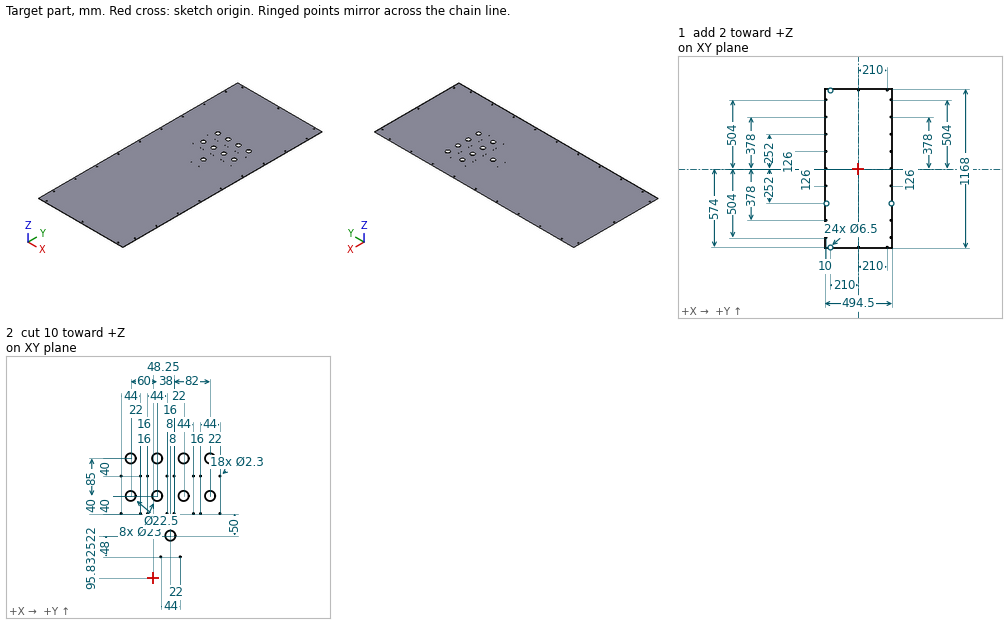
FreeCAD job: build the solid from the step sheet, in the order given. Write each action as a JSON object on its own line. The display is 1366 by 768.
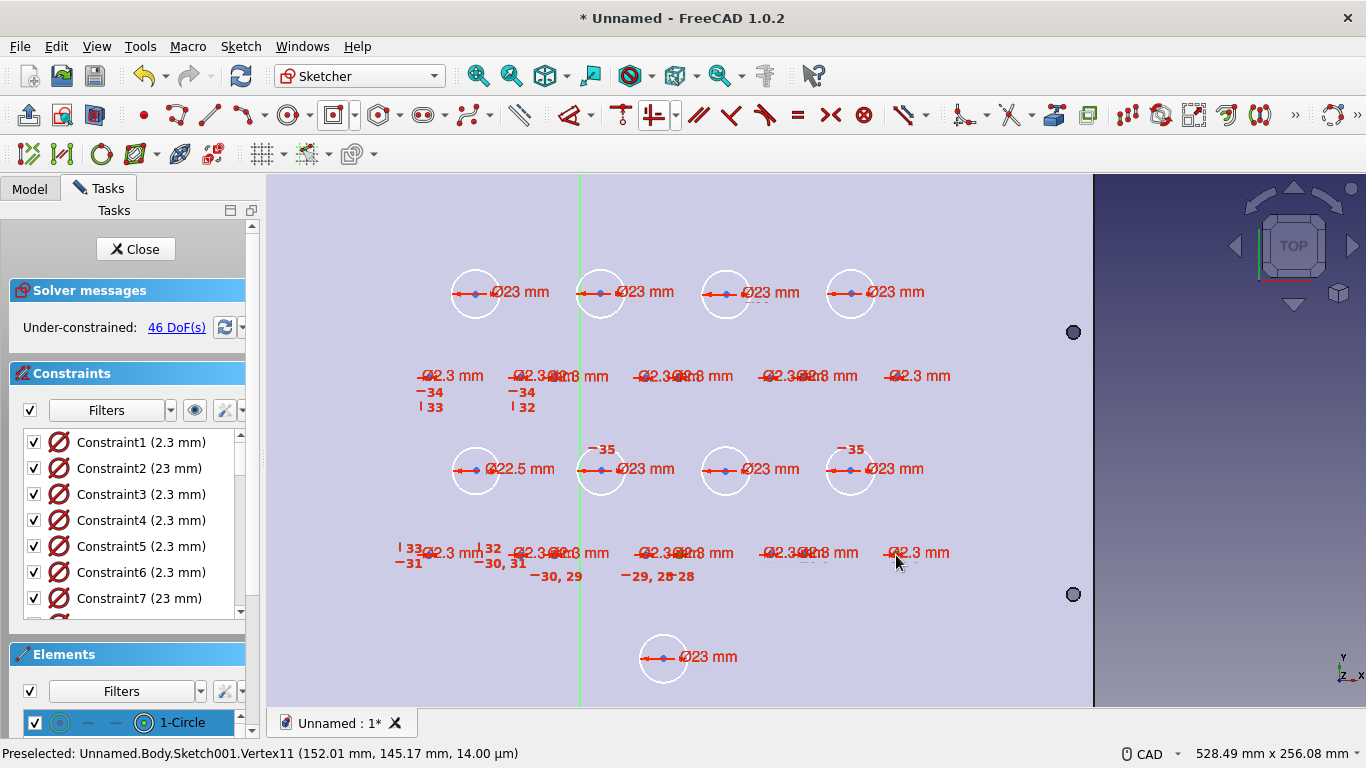
{"action": "left_click", "coordinate": [676, 116]}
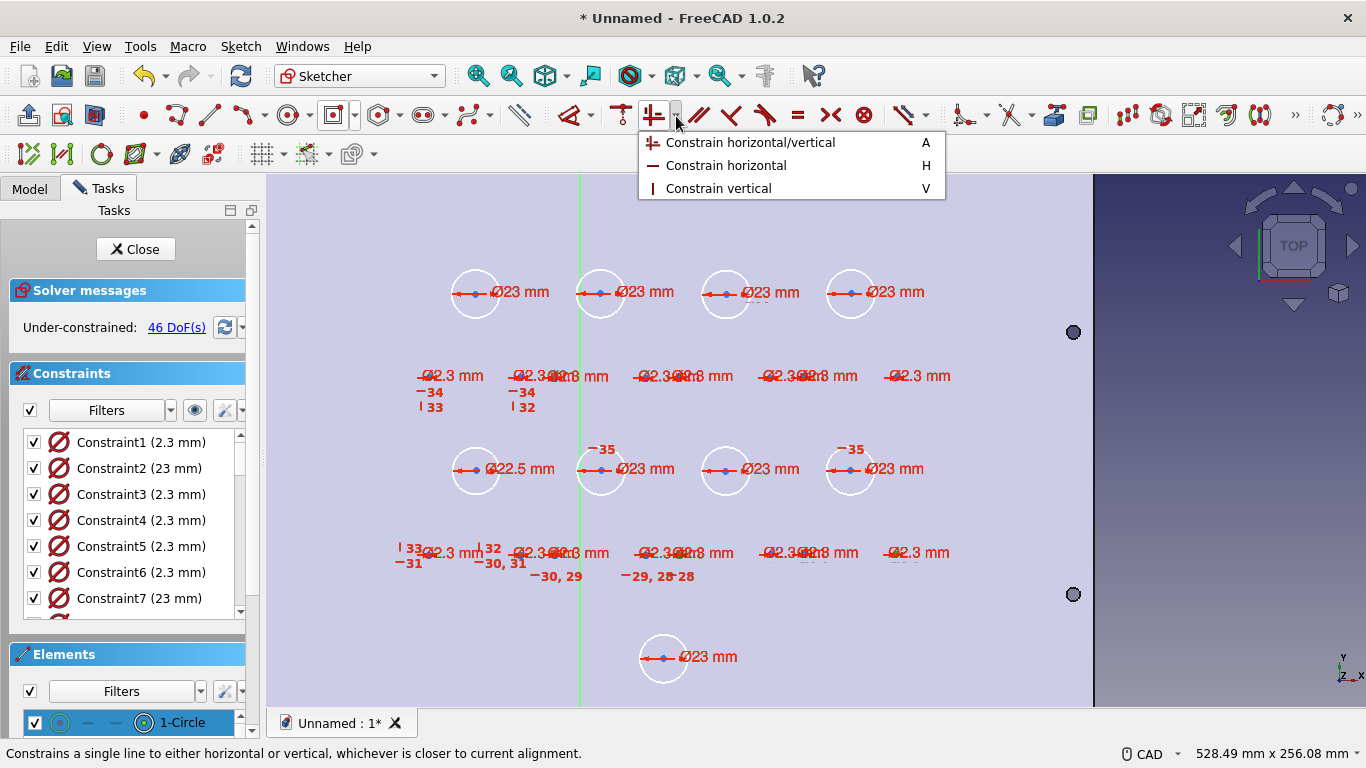
{"action": "left_click", "coordinate": [792, 166]}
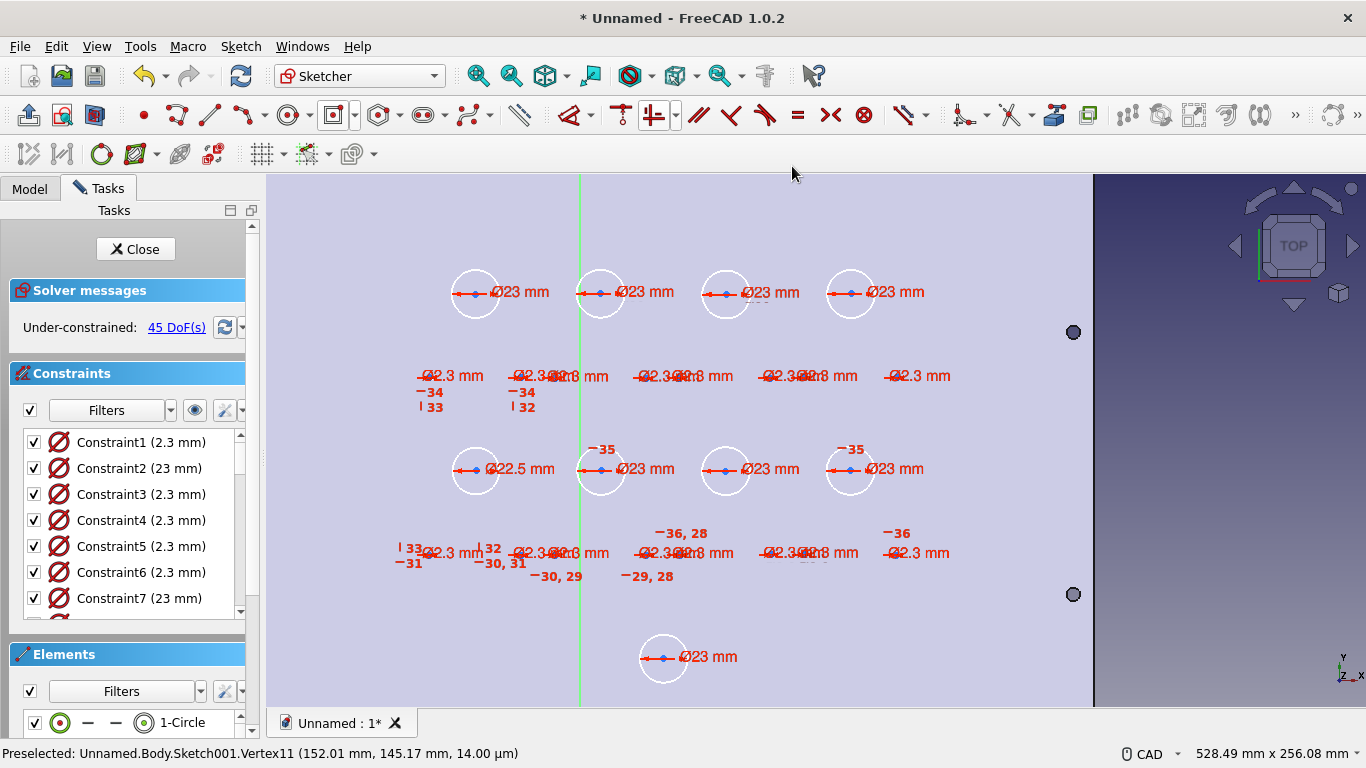
{"action": "left_click", "coordinate": [896, 555]}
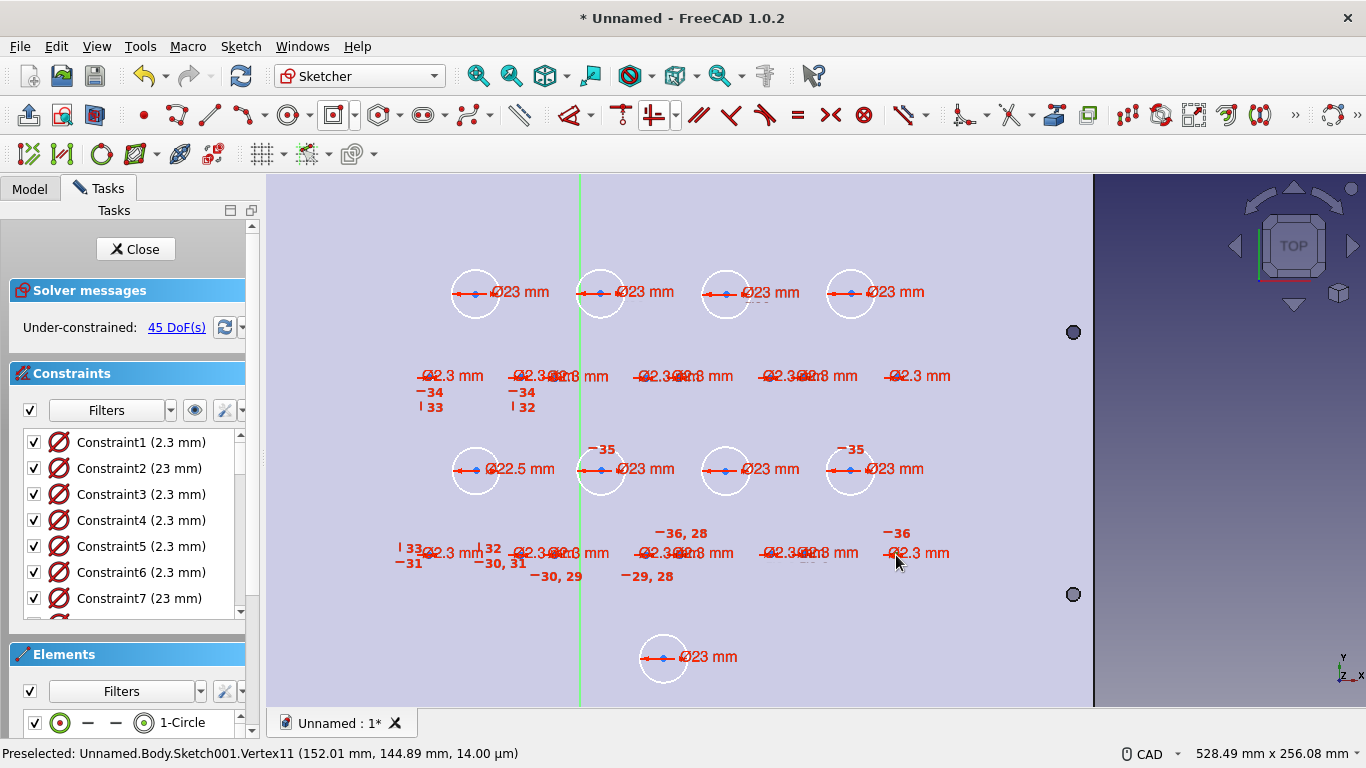
{"action": "left_click", "coordinate": [805, 555]}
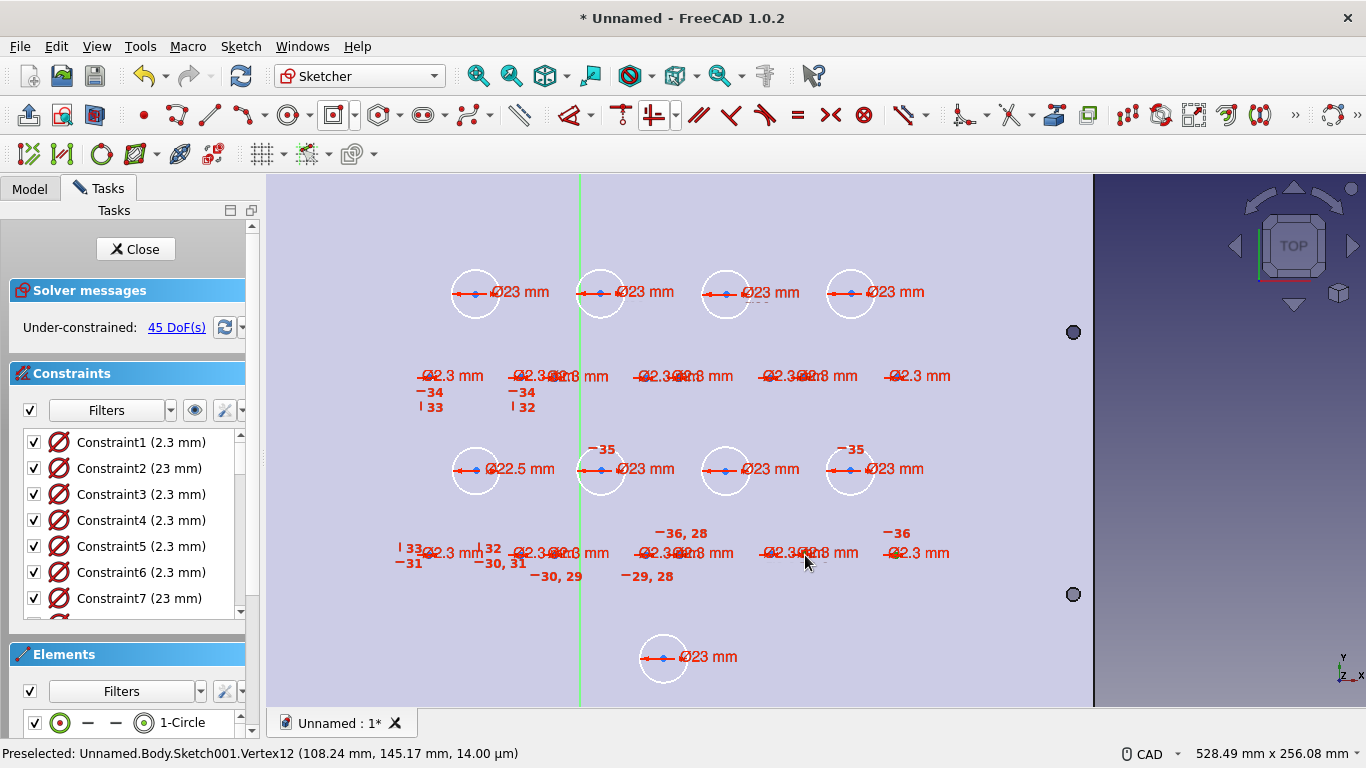
{"action": "left_click", "coordinate": [676, 116]}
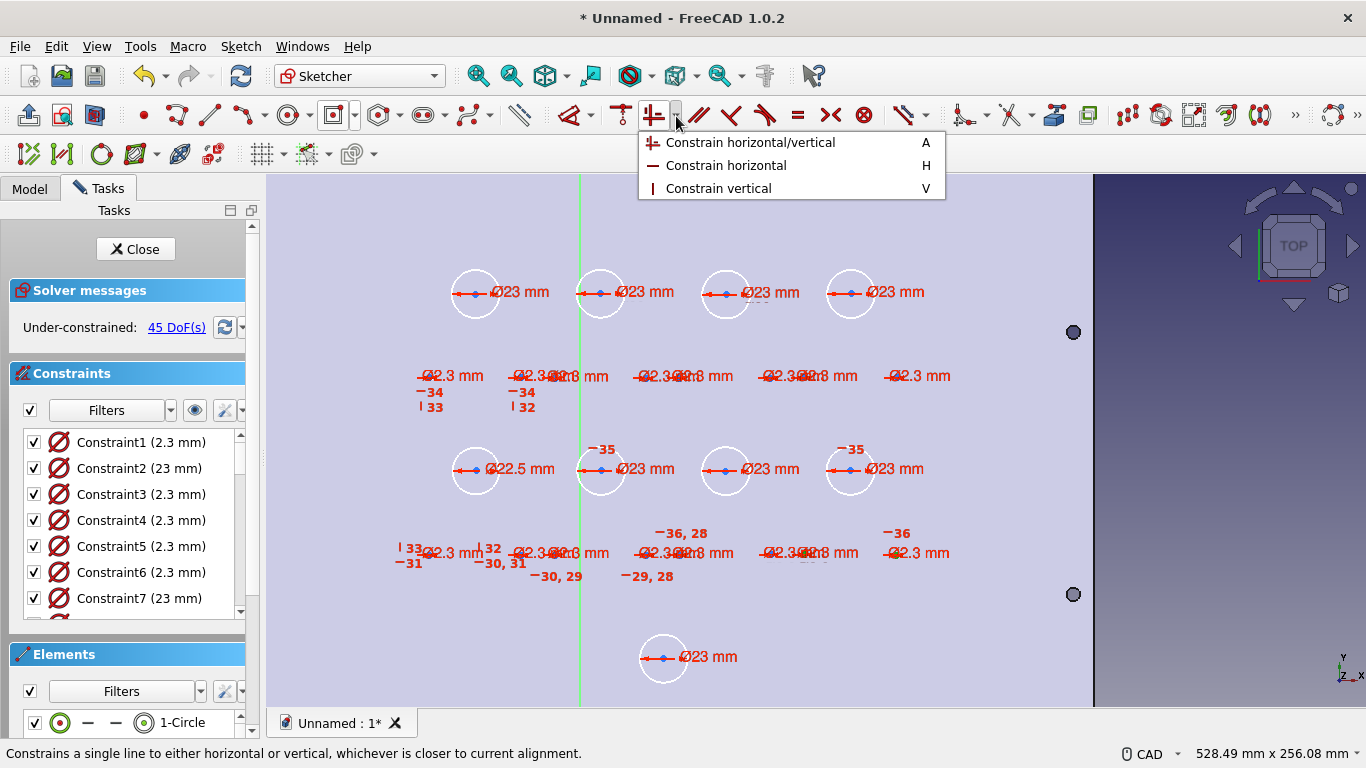
{"action": "left_click", "coordinate": [792, 166]}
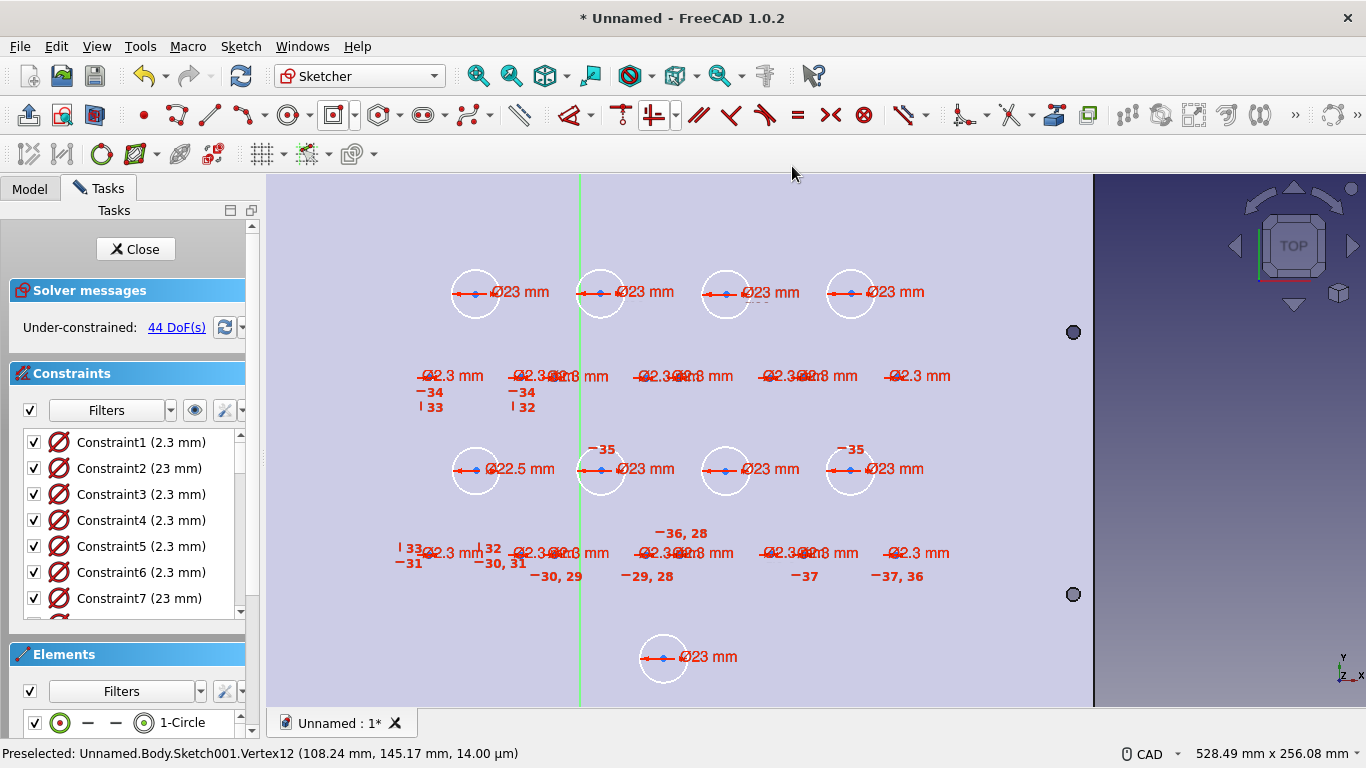
{"action": "left_click", "coordinate": [601, 471]}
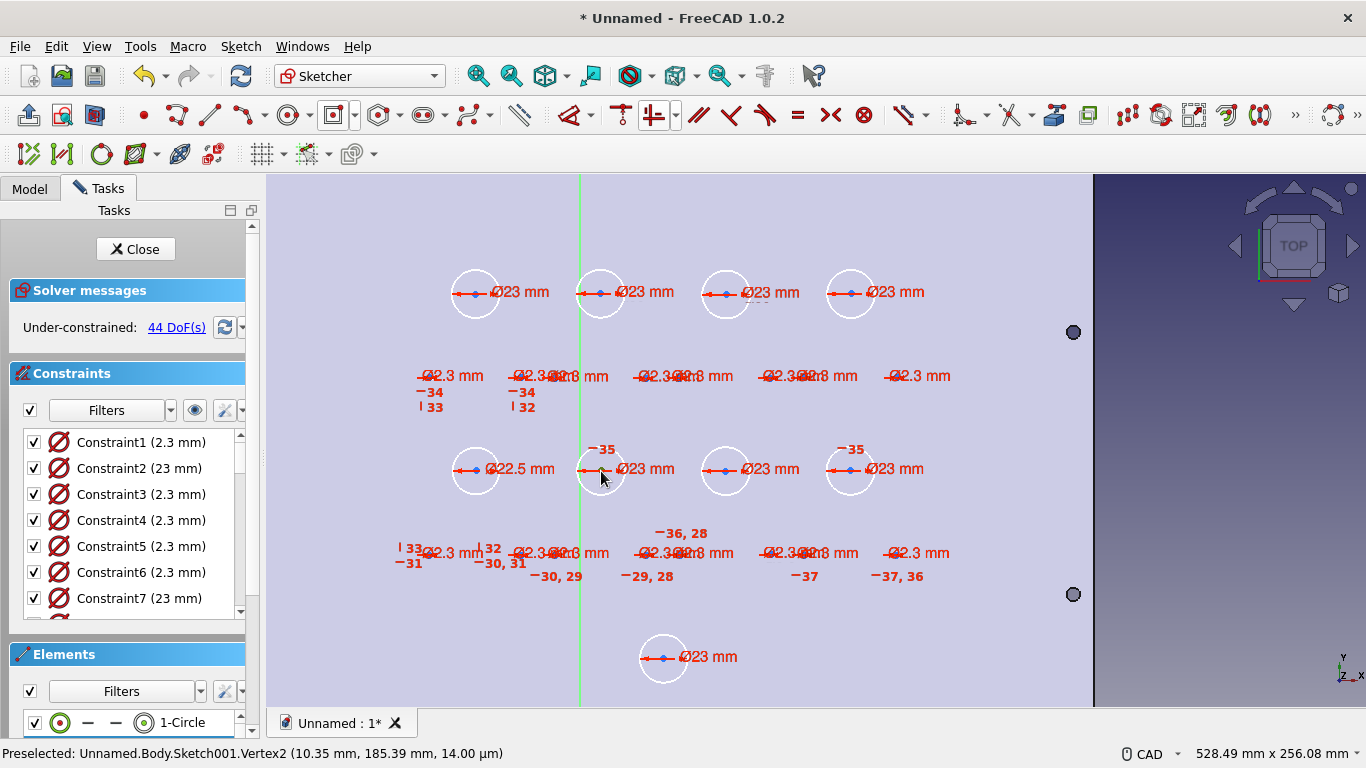
{"action": "left_click", "coordinate": [726, 471]}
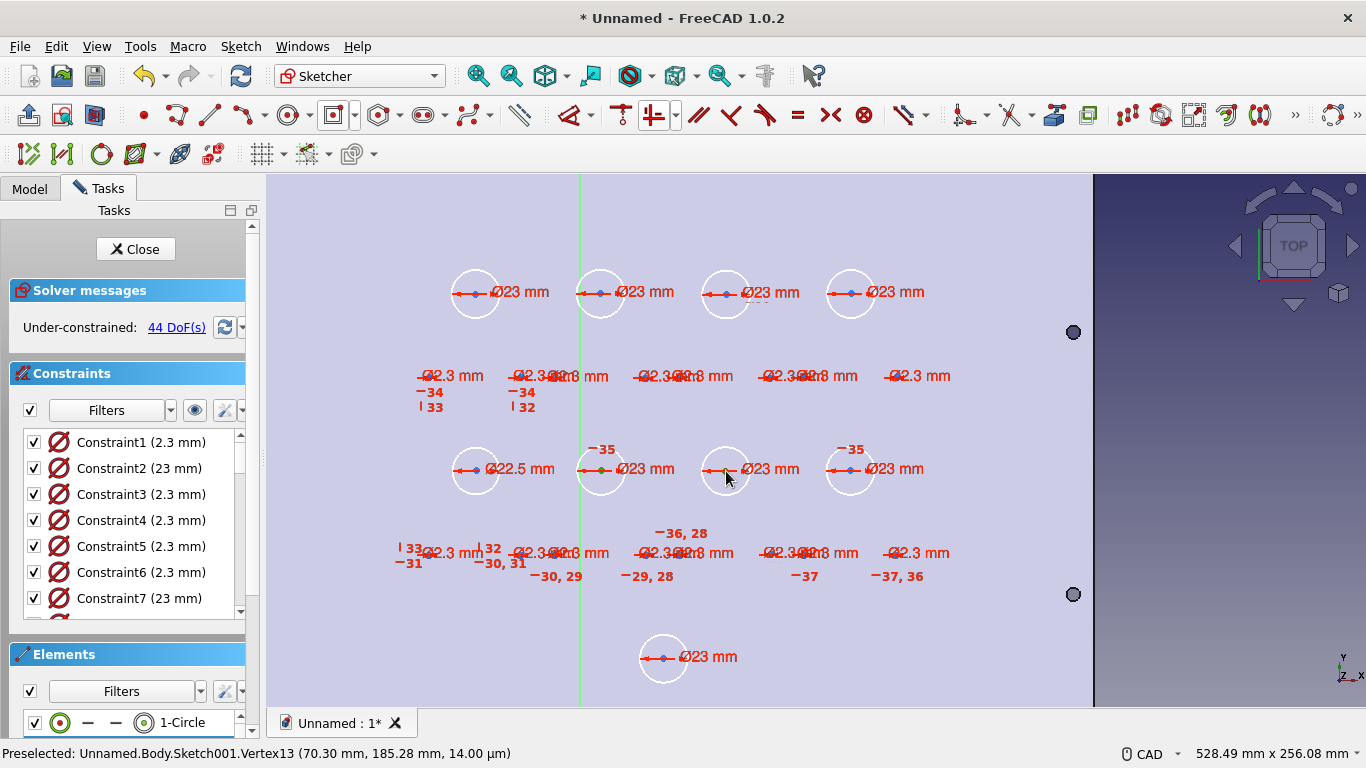
{"action": "left_click", "coordinate": [676, 116]}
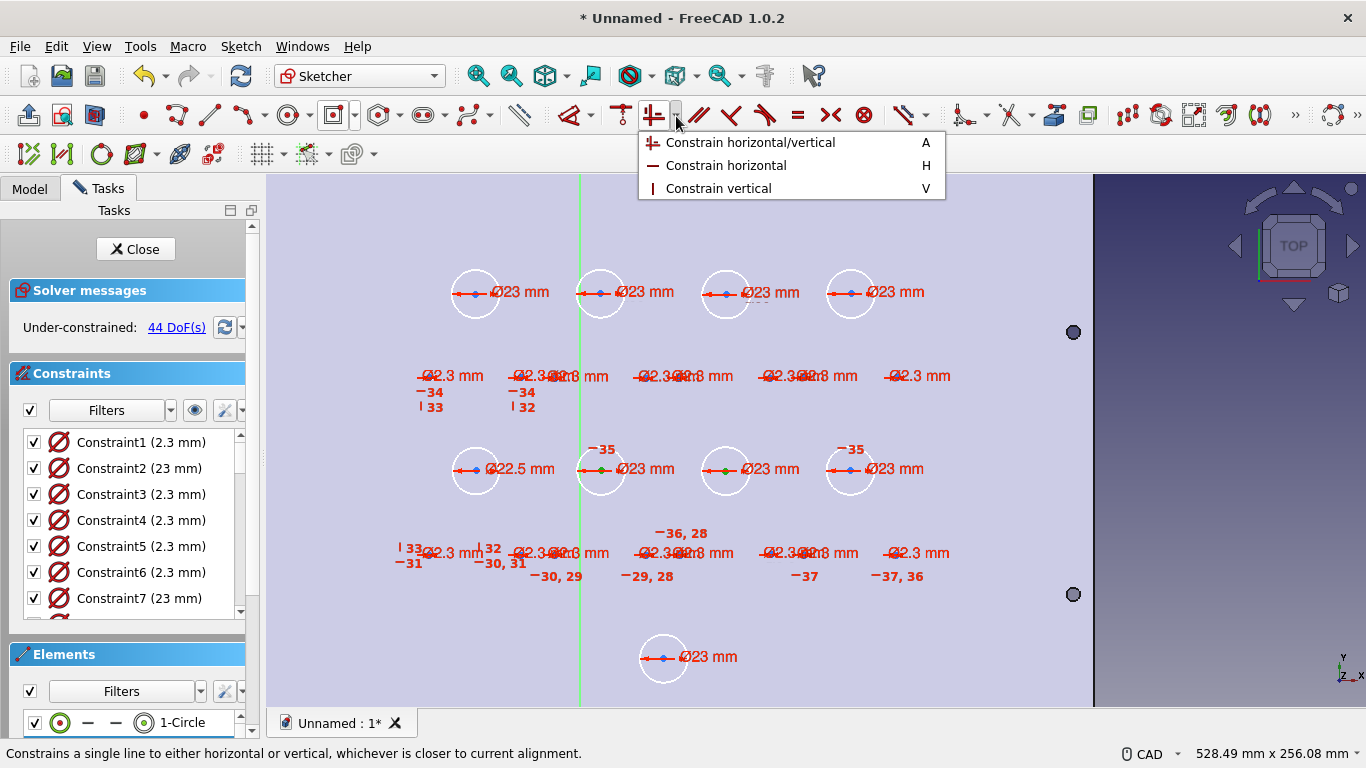
{"action": "left_click", "coordinate": [792, 166]}